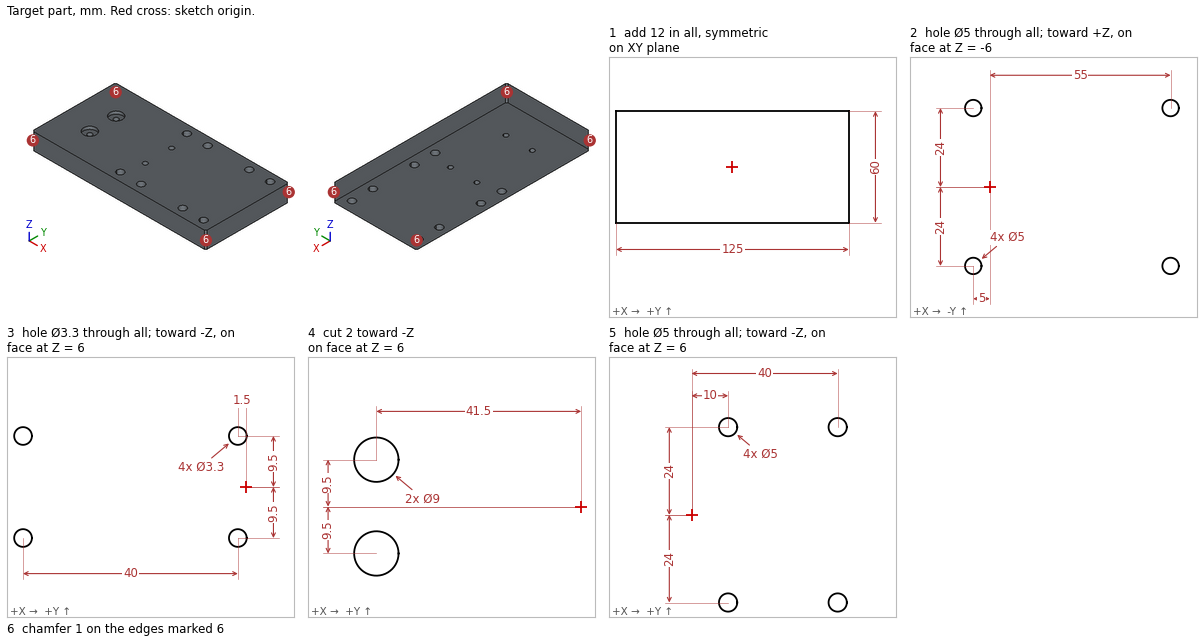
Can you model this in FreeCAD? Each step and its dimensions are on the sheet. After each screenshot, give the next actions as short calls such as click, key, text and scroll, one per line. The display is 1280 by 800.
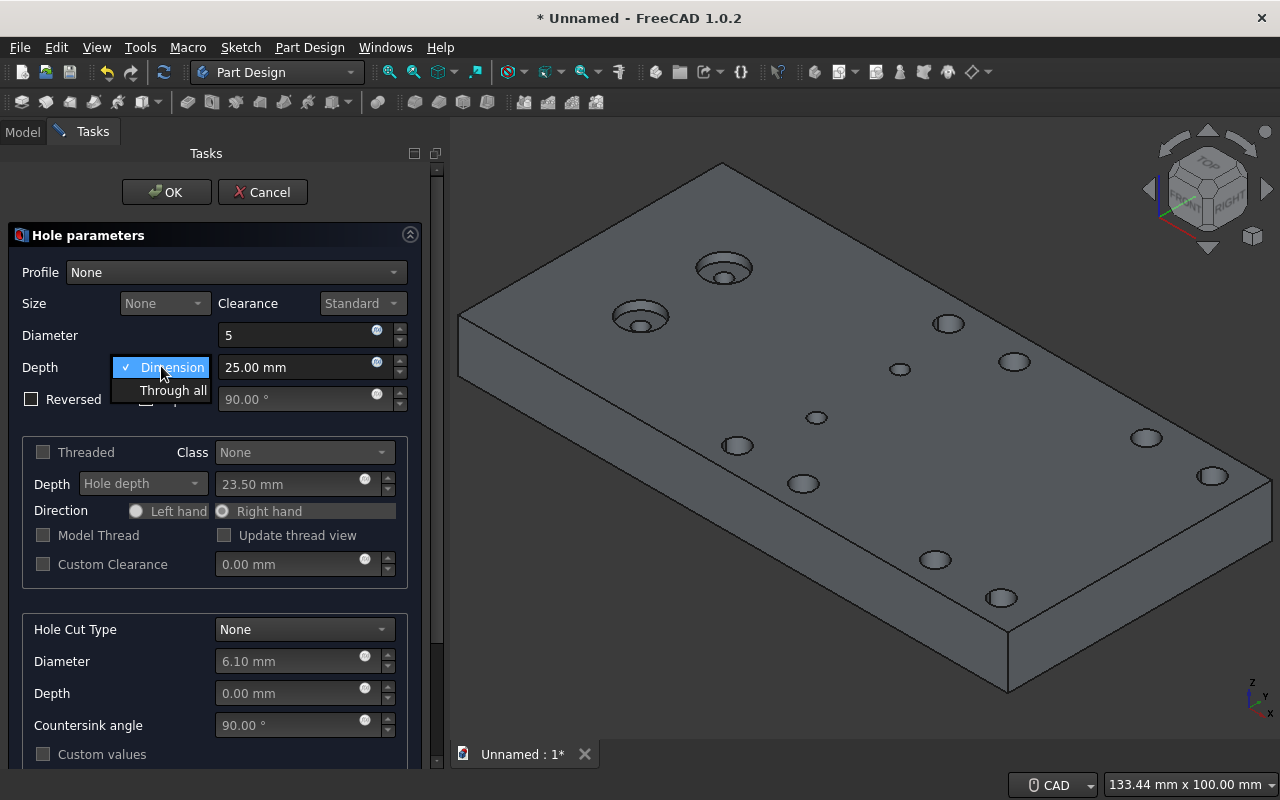
click(160, 390)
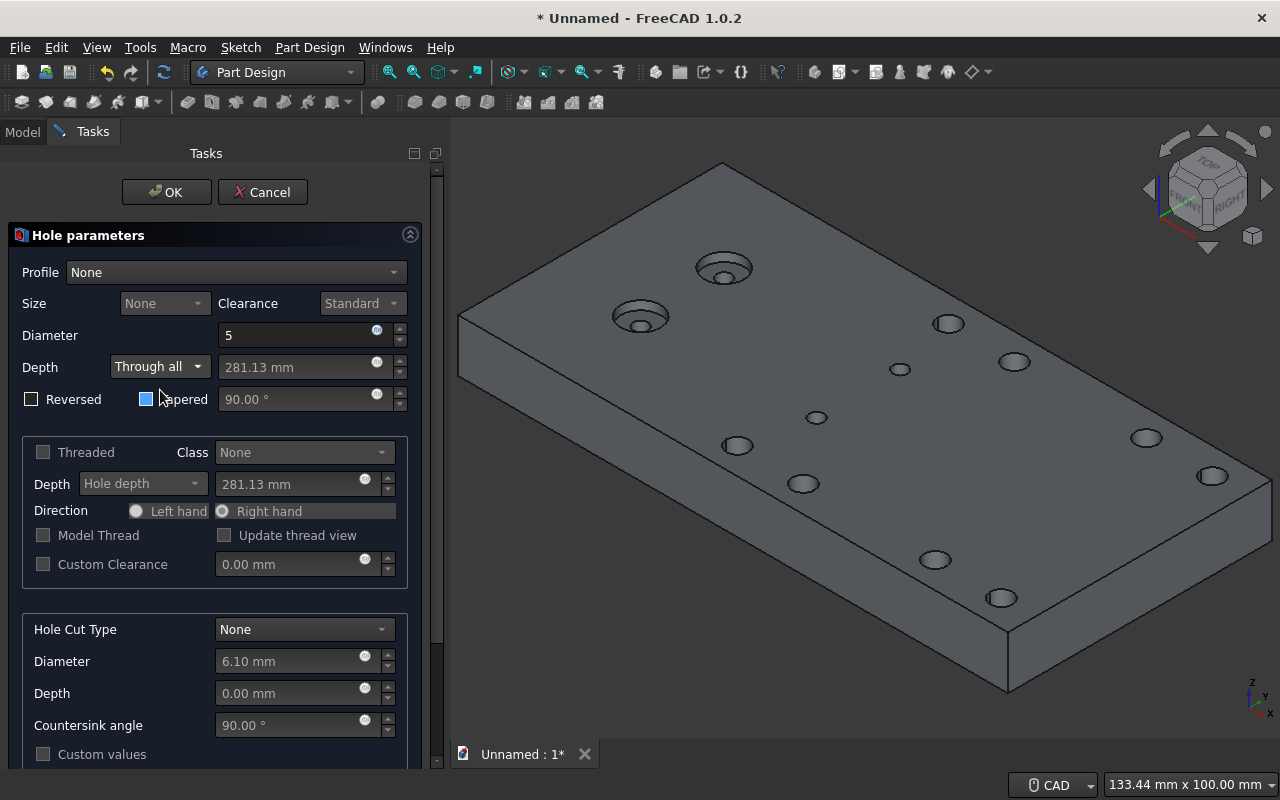
click(167, 192)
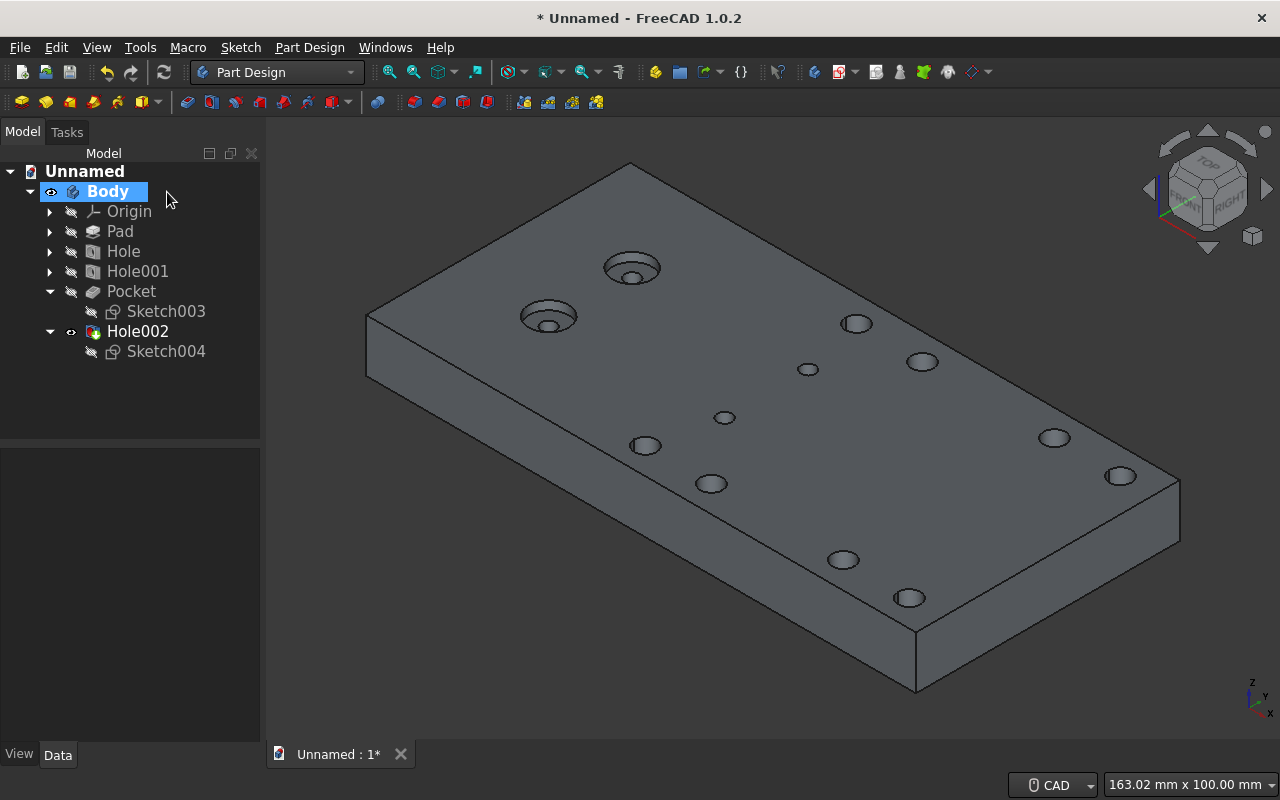
click(916, 662)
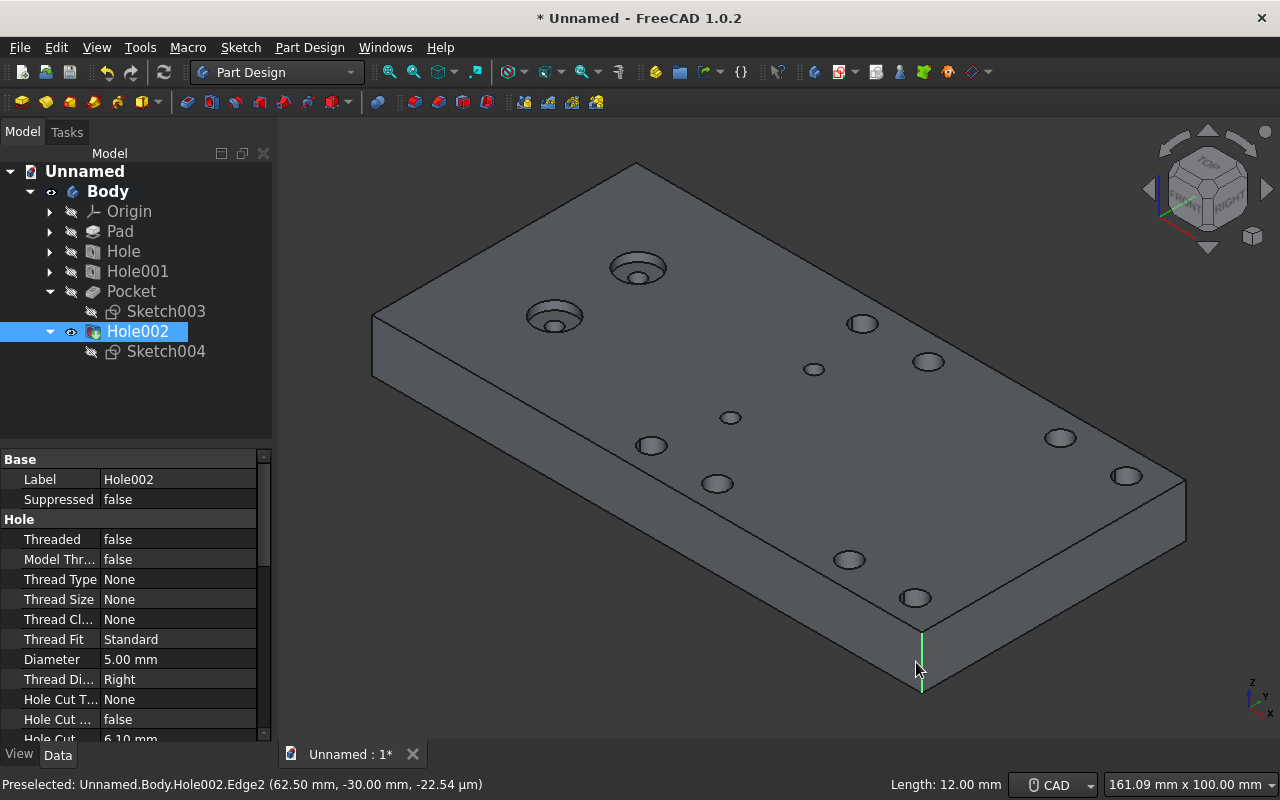
key(2)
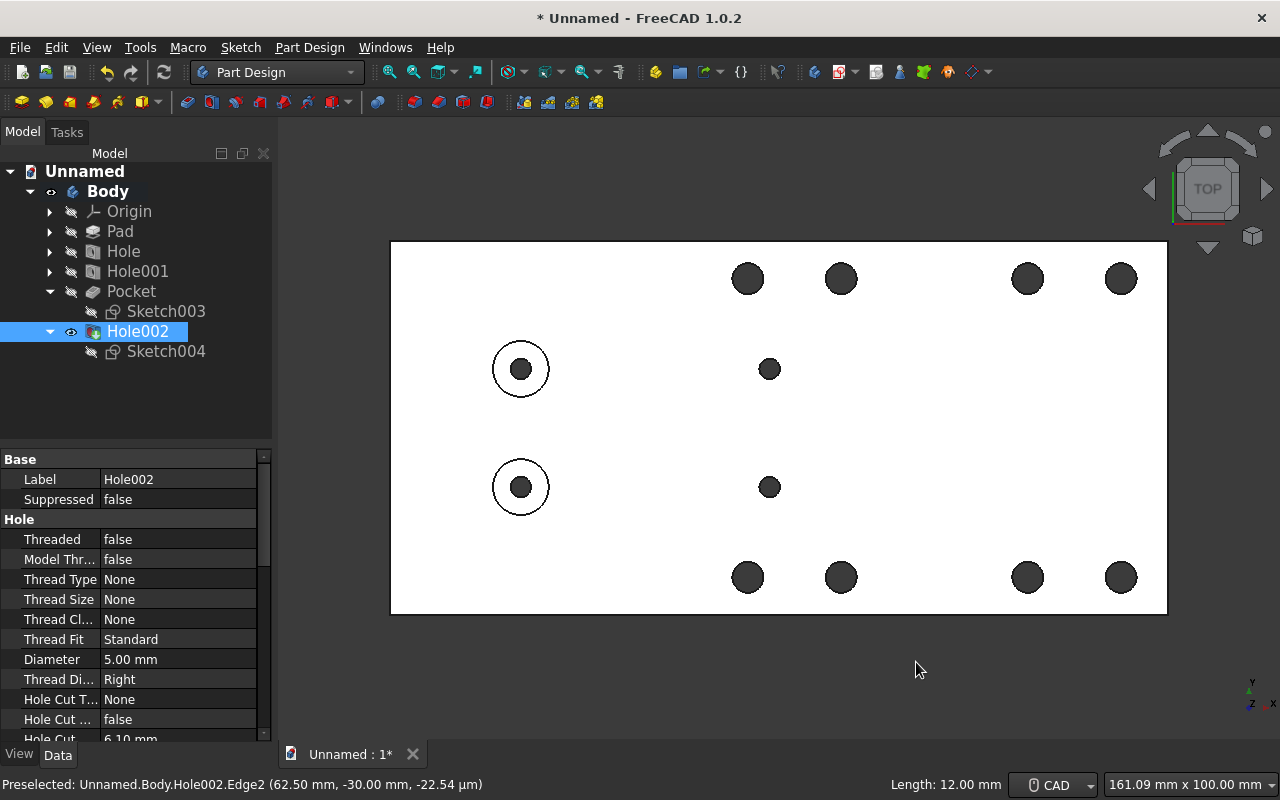
key(0)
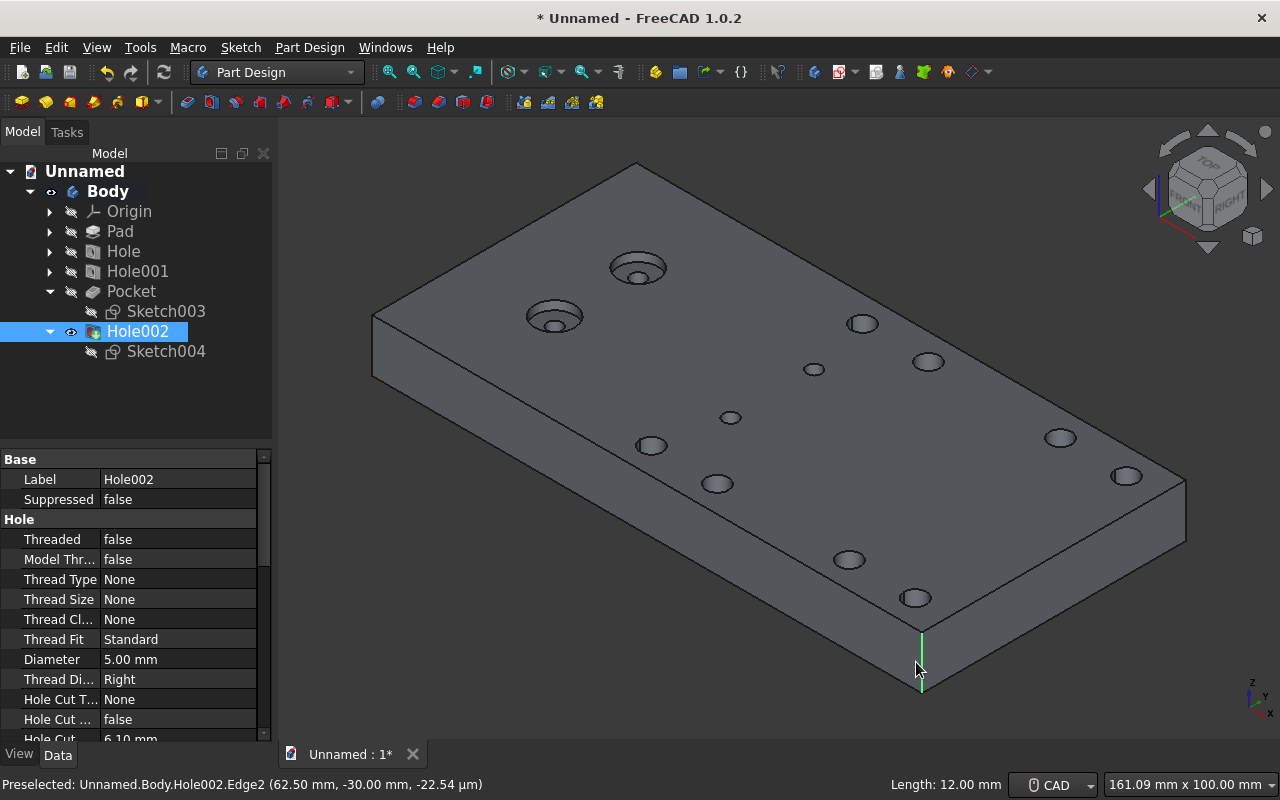
key(1)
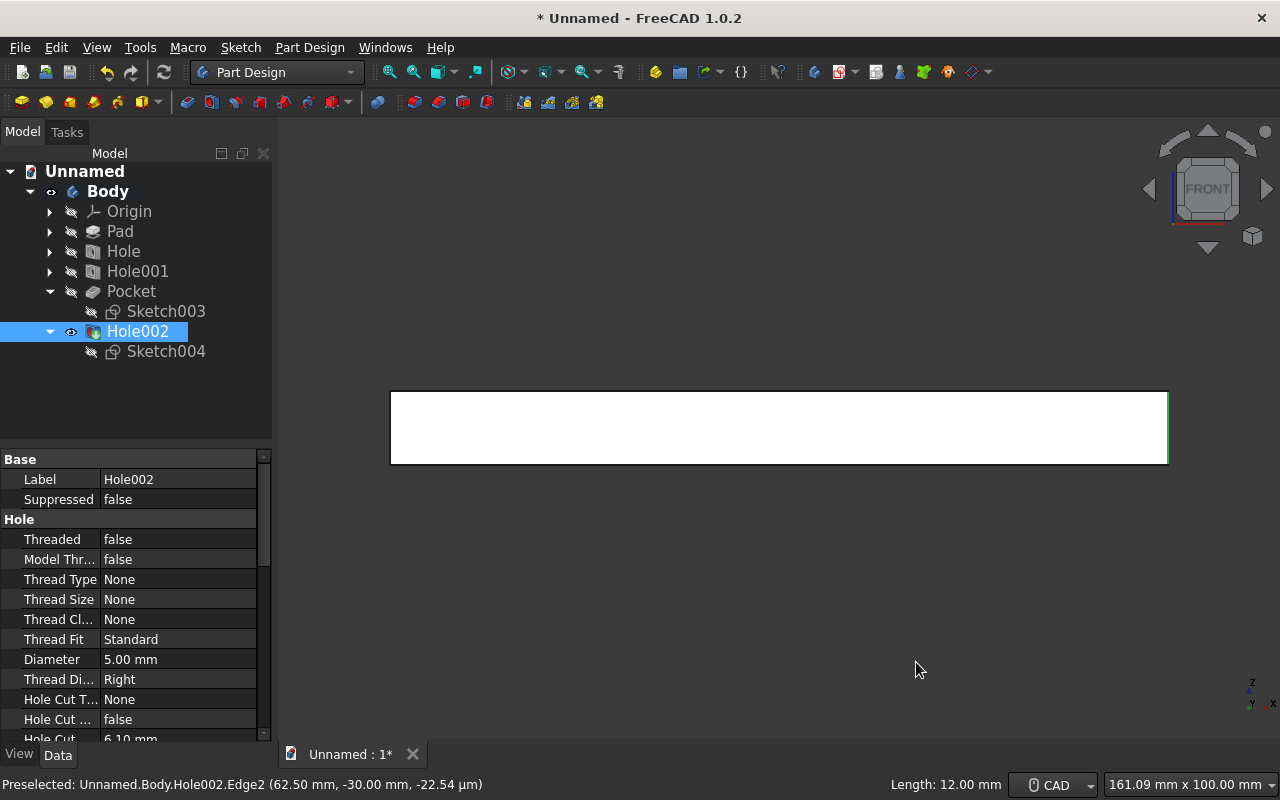
click(390, 427, ctrl)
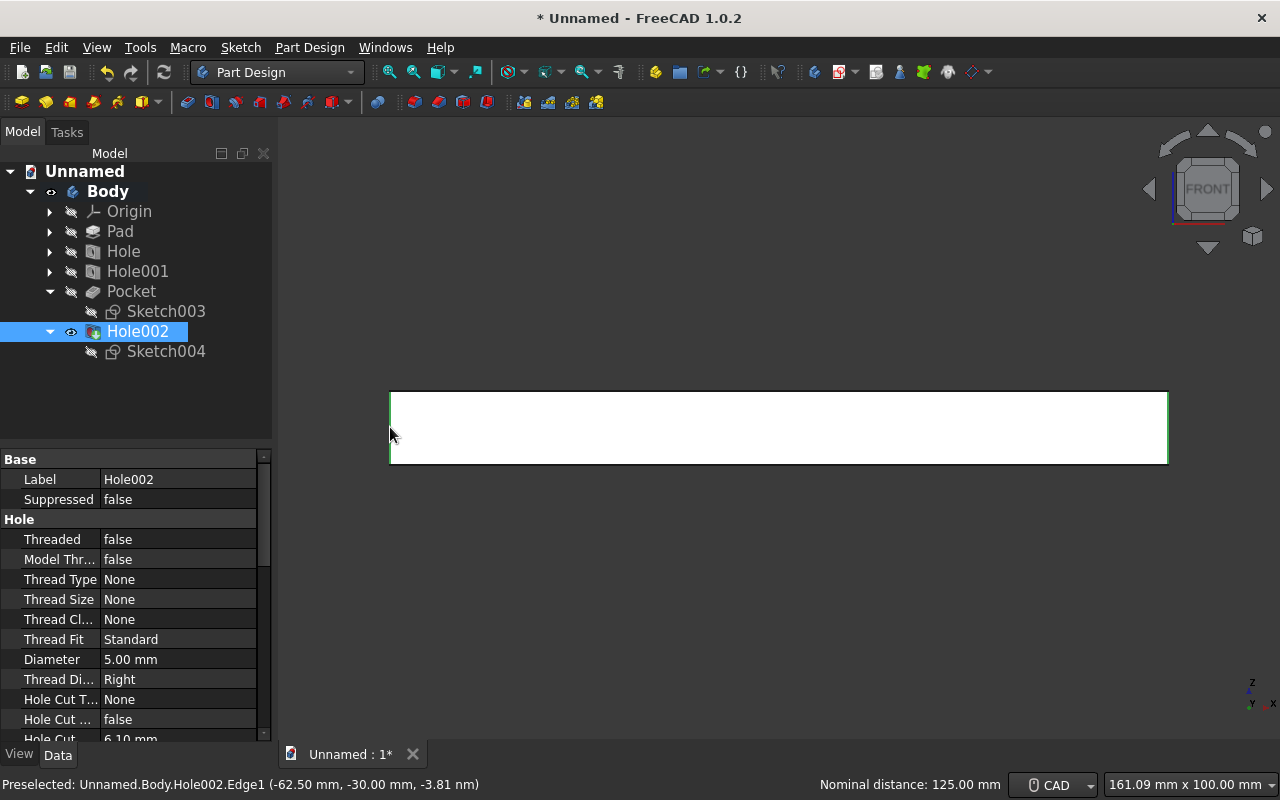
key(3)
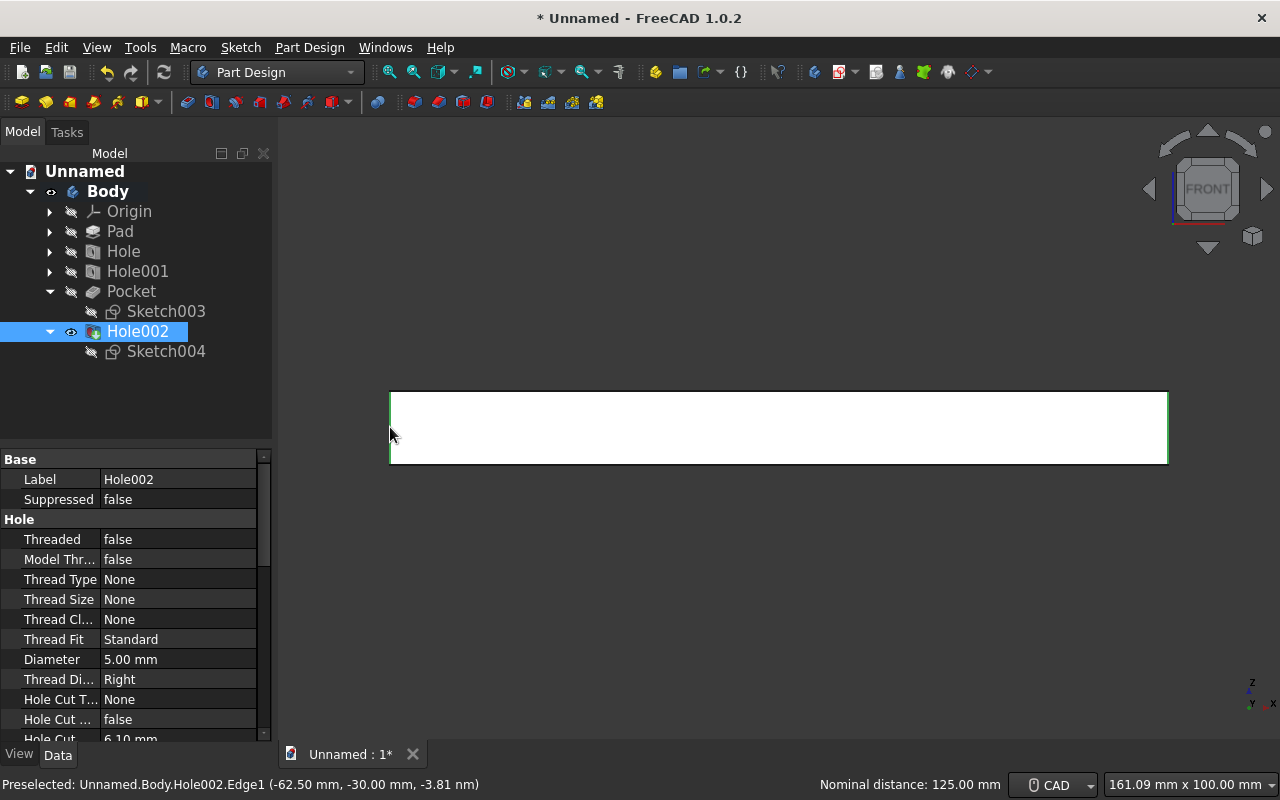
key(v)
key(f)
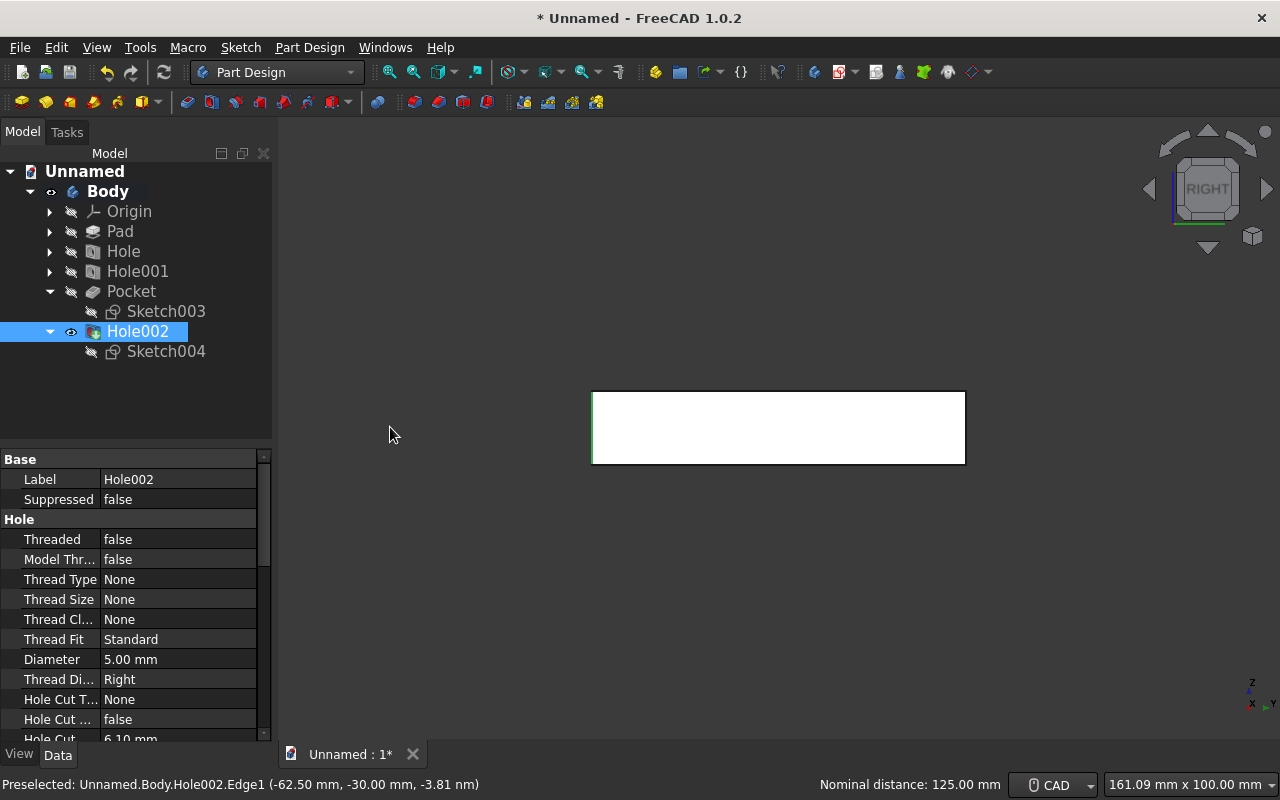
click(913, 427, ctrl)